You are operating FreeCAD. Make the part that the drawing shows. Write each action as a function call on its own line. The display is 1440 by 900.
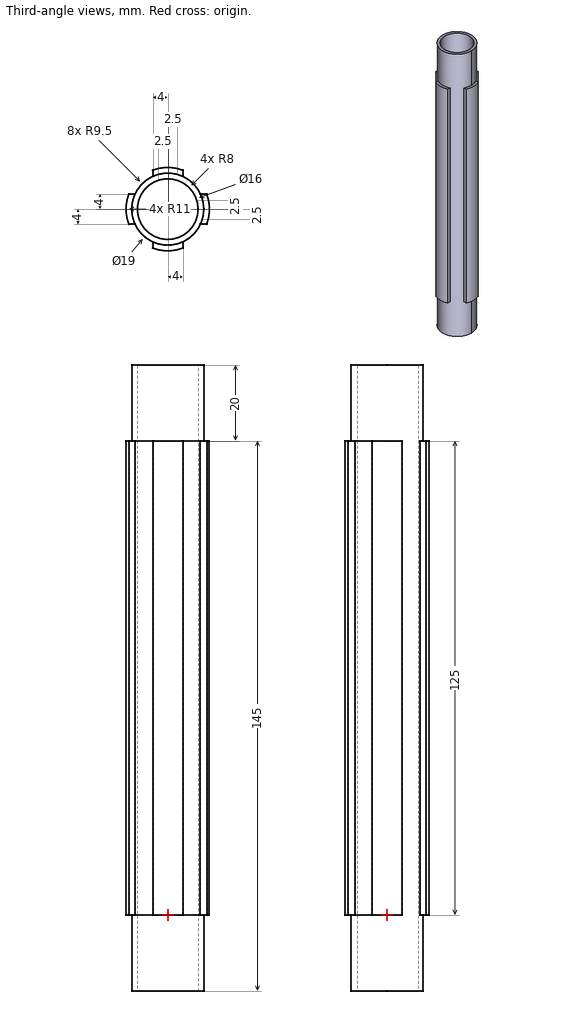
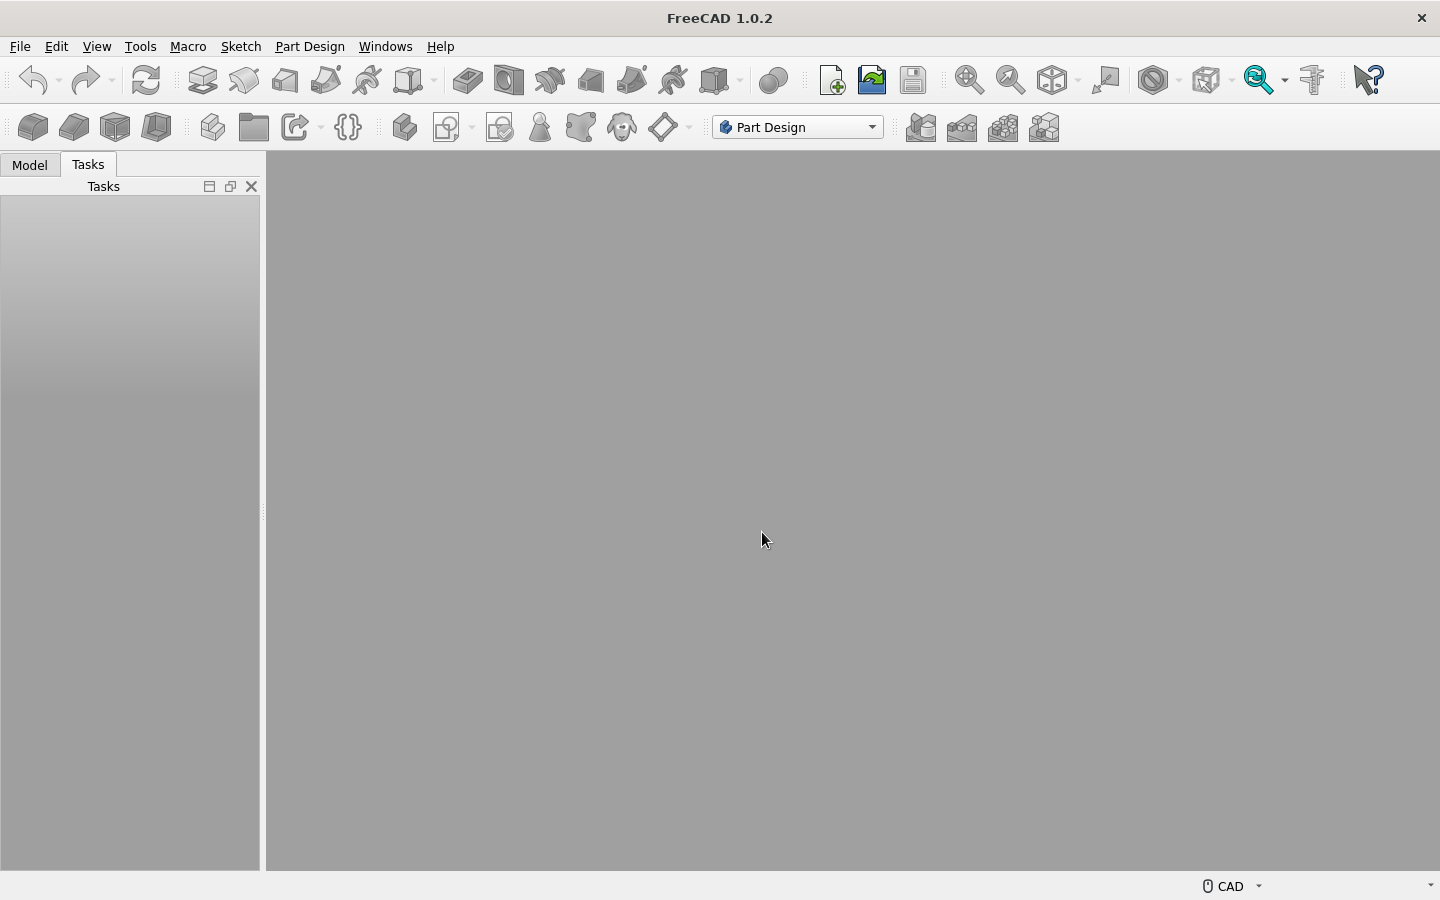
click(831, 80)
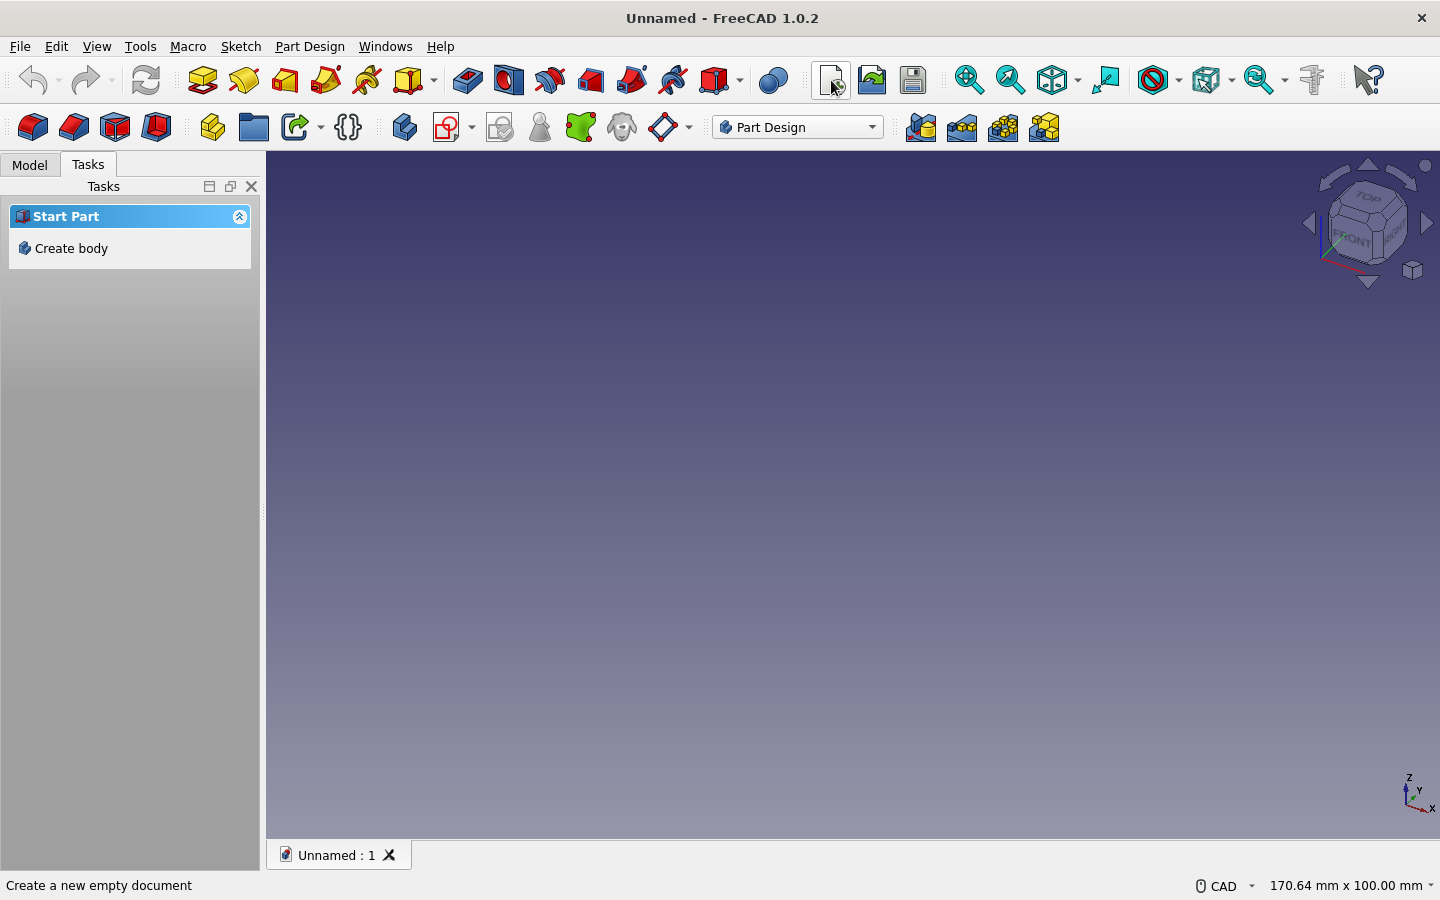
click(446, 128)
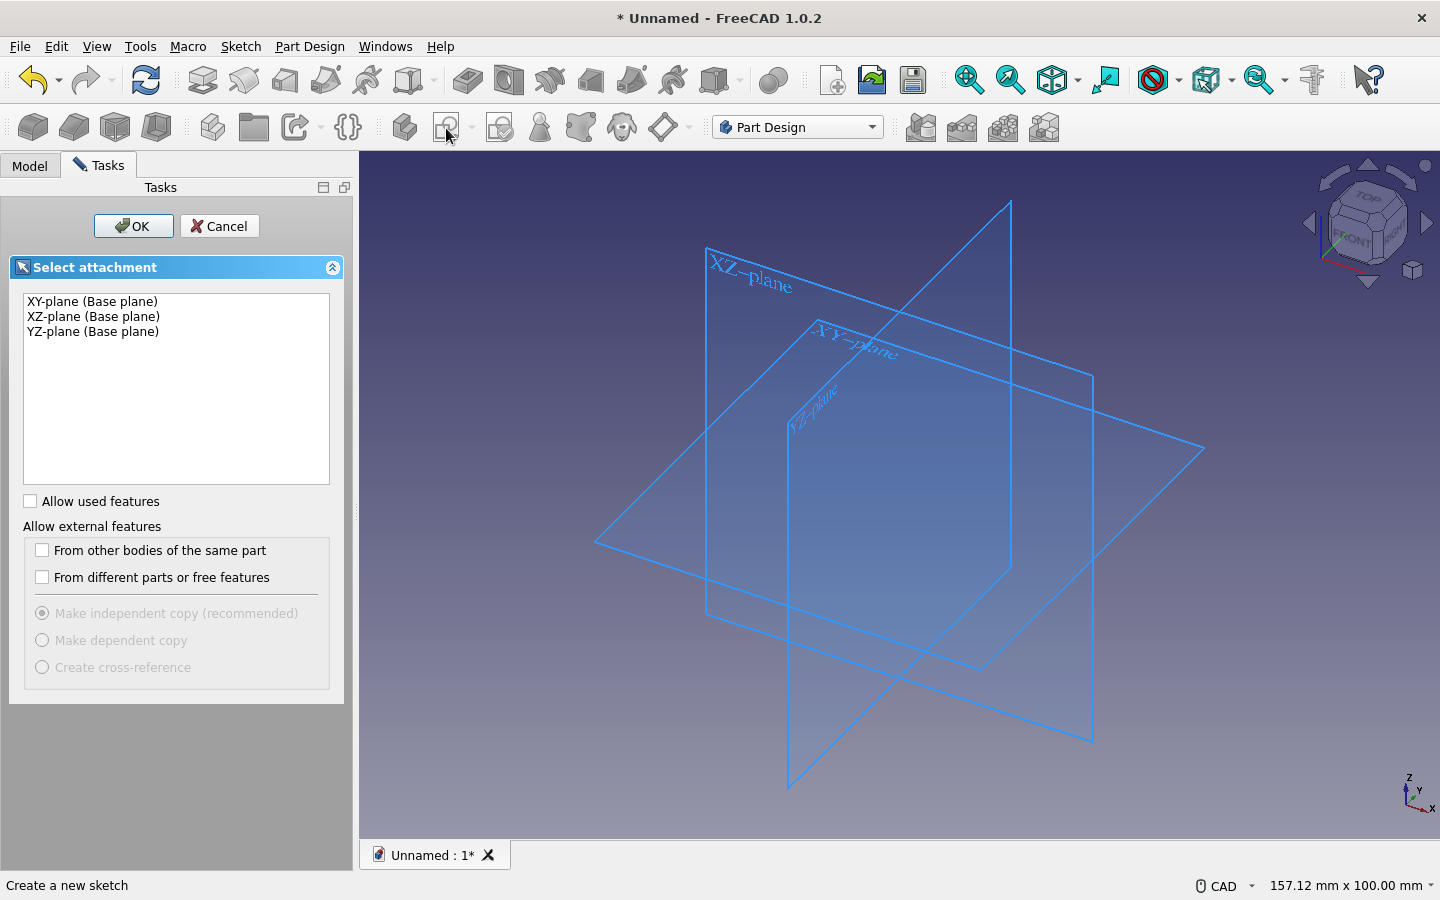
click(84, 302)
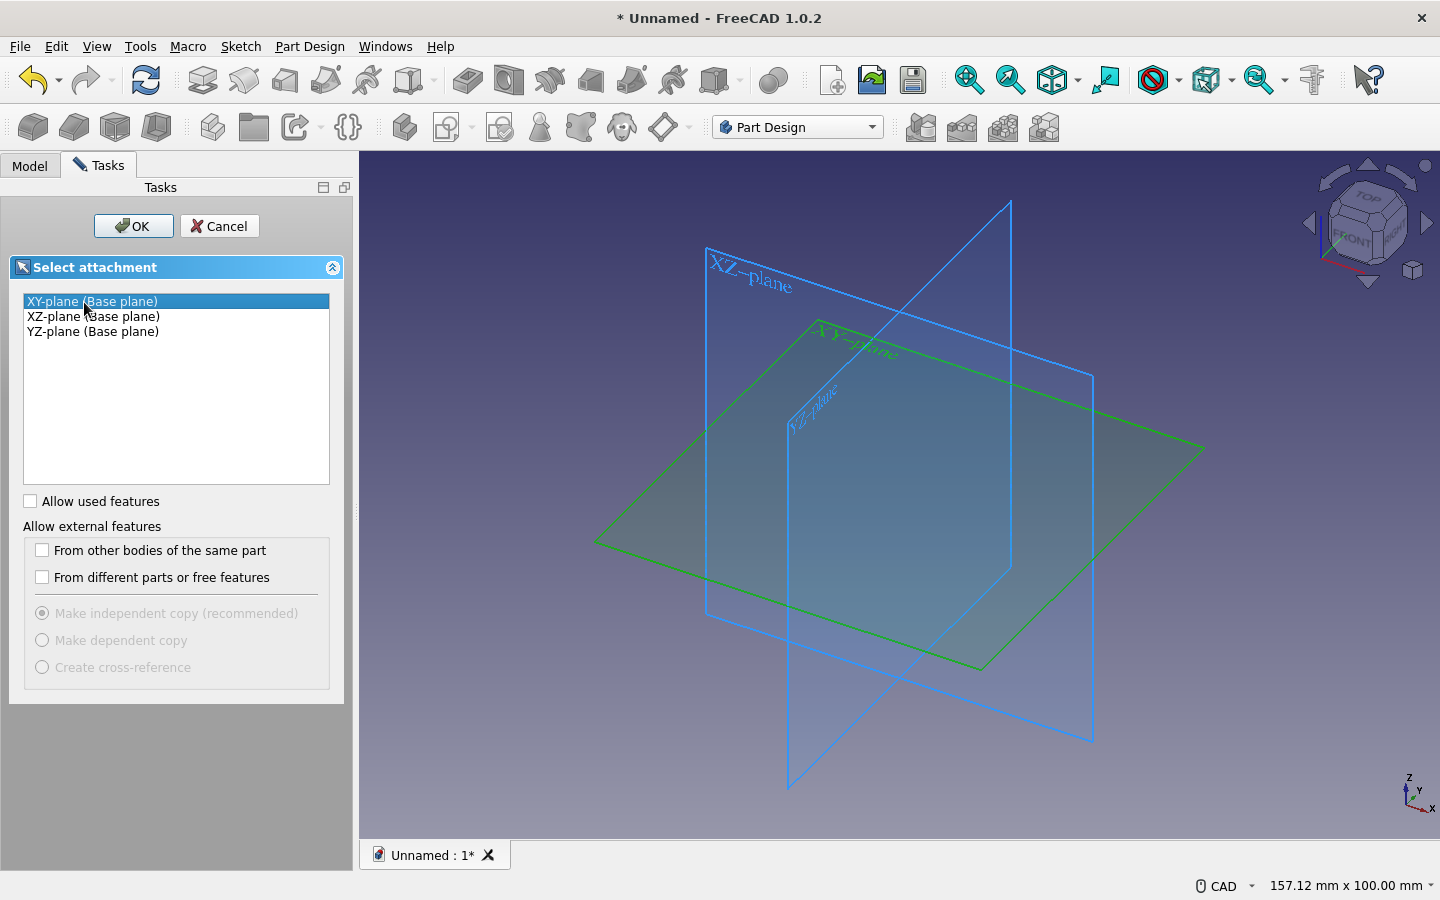
click(134, 226)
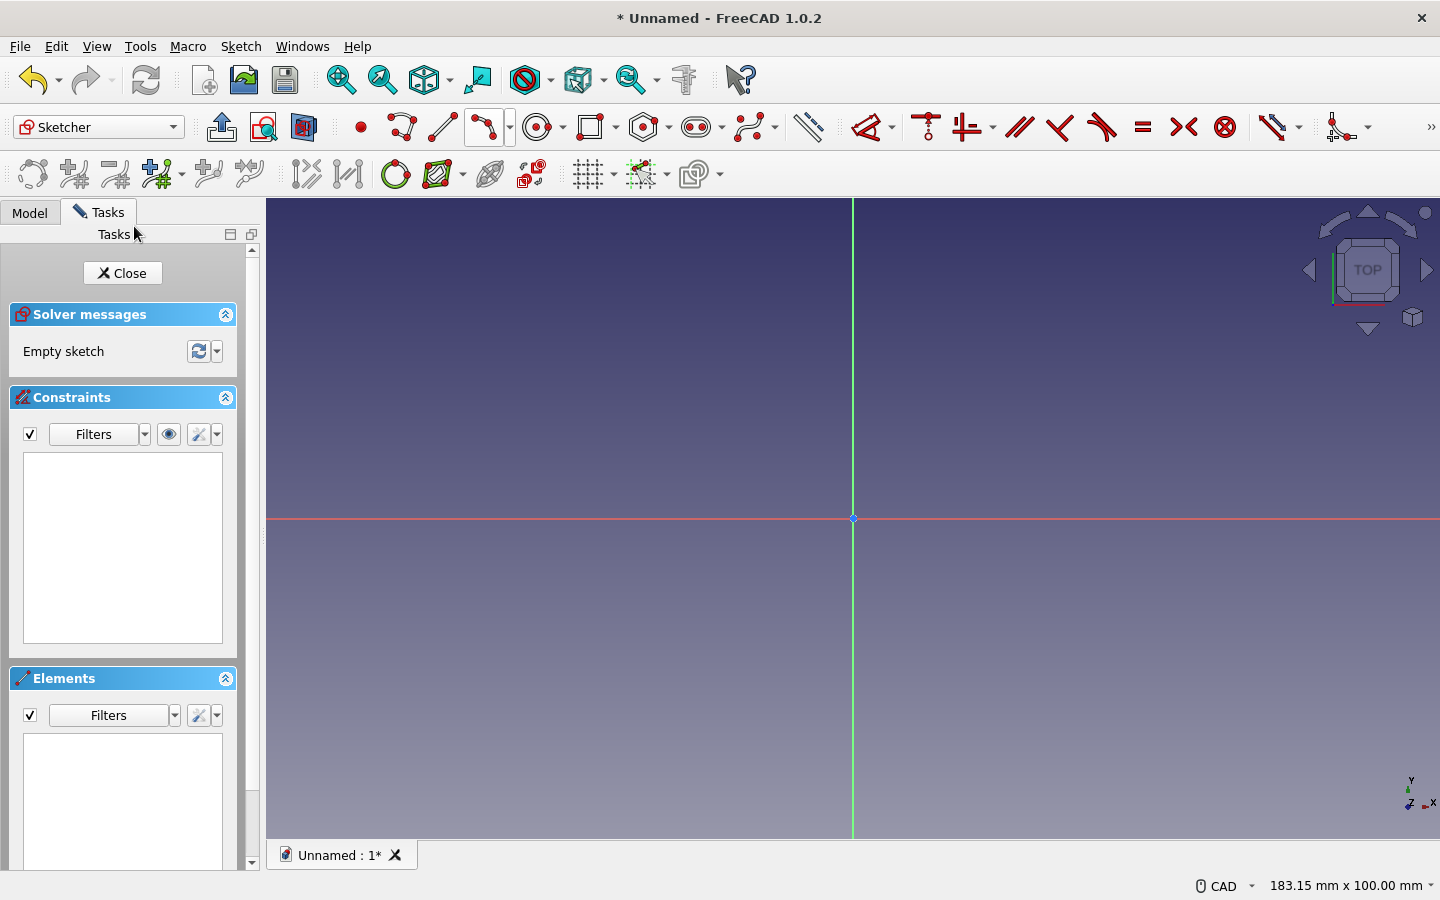
scroll(893, 518, up, 5)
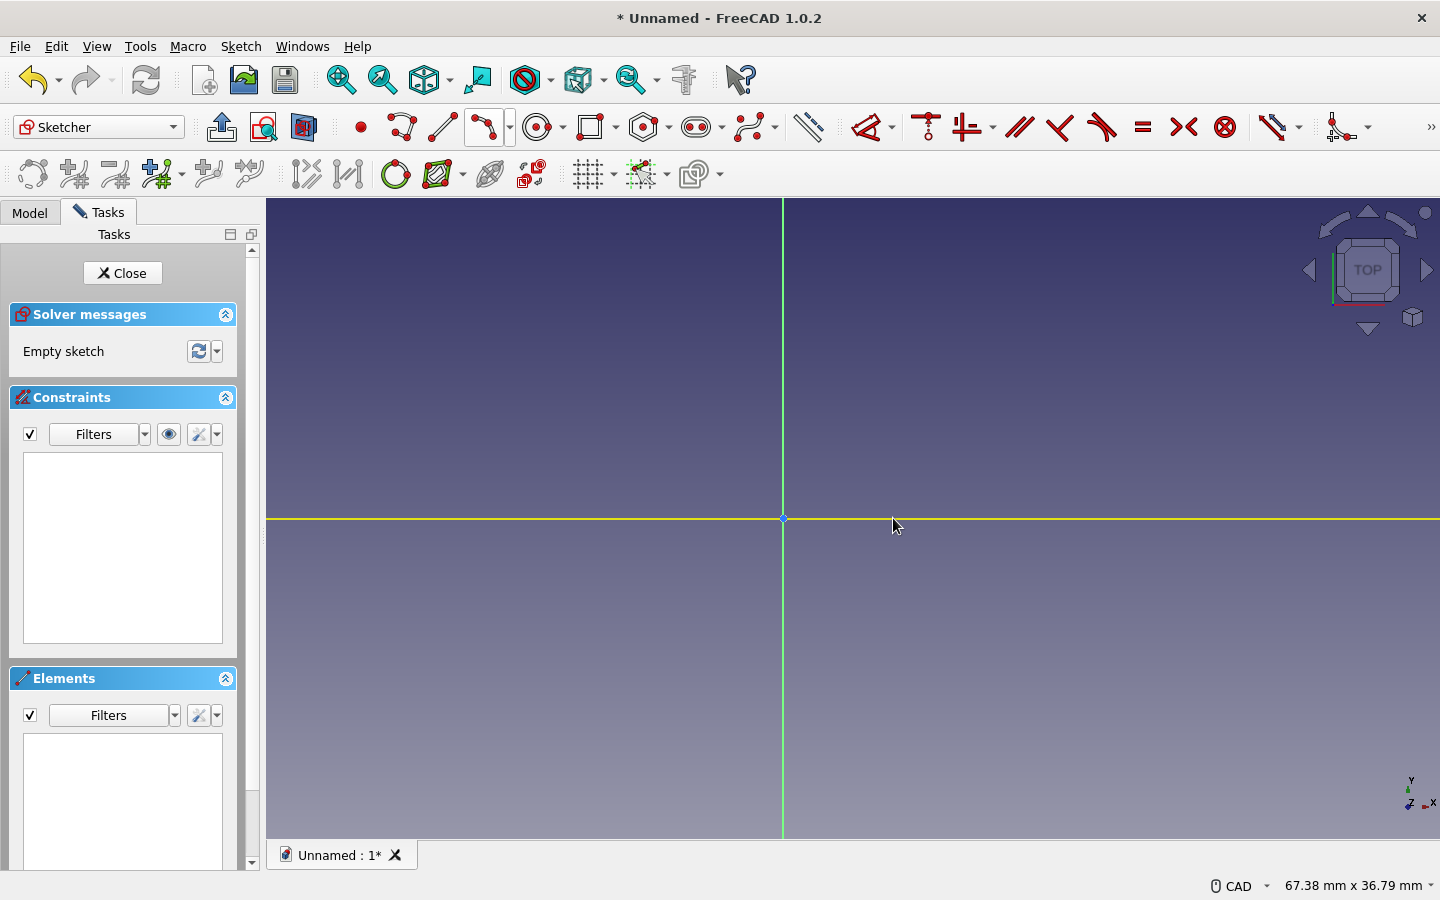
click(443, 128)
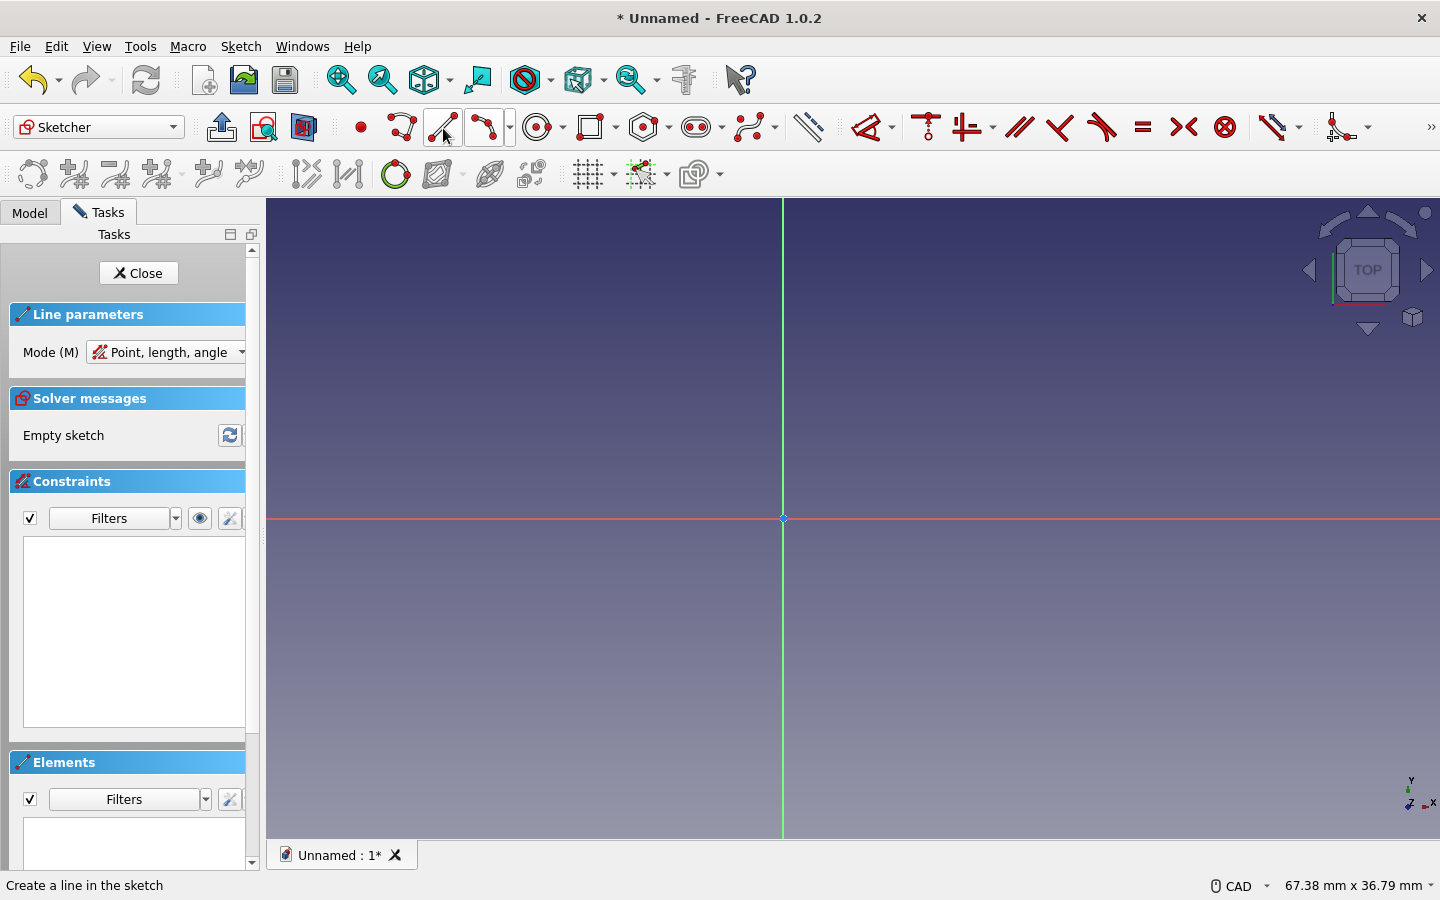
click(714, 340)
click(714, 368)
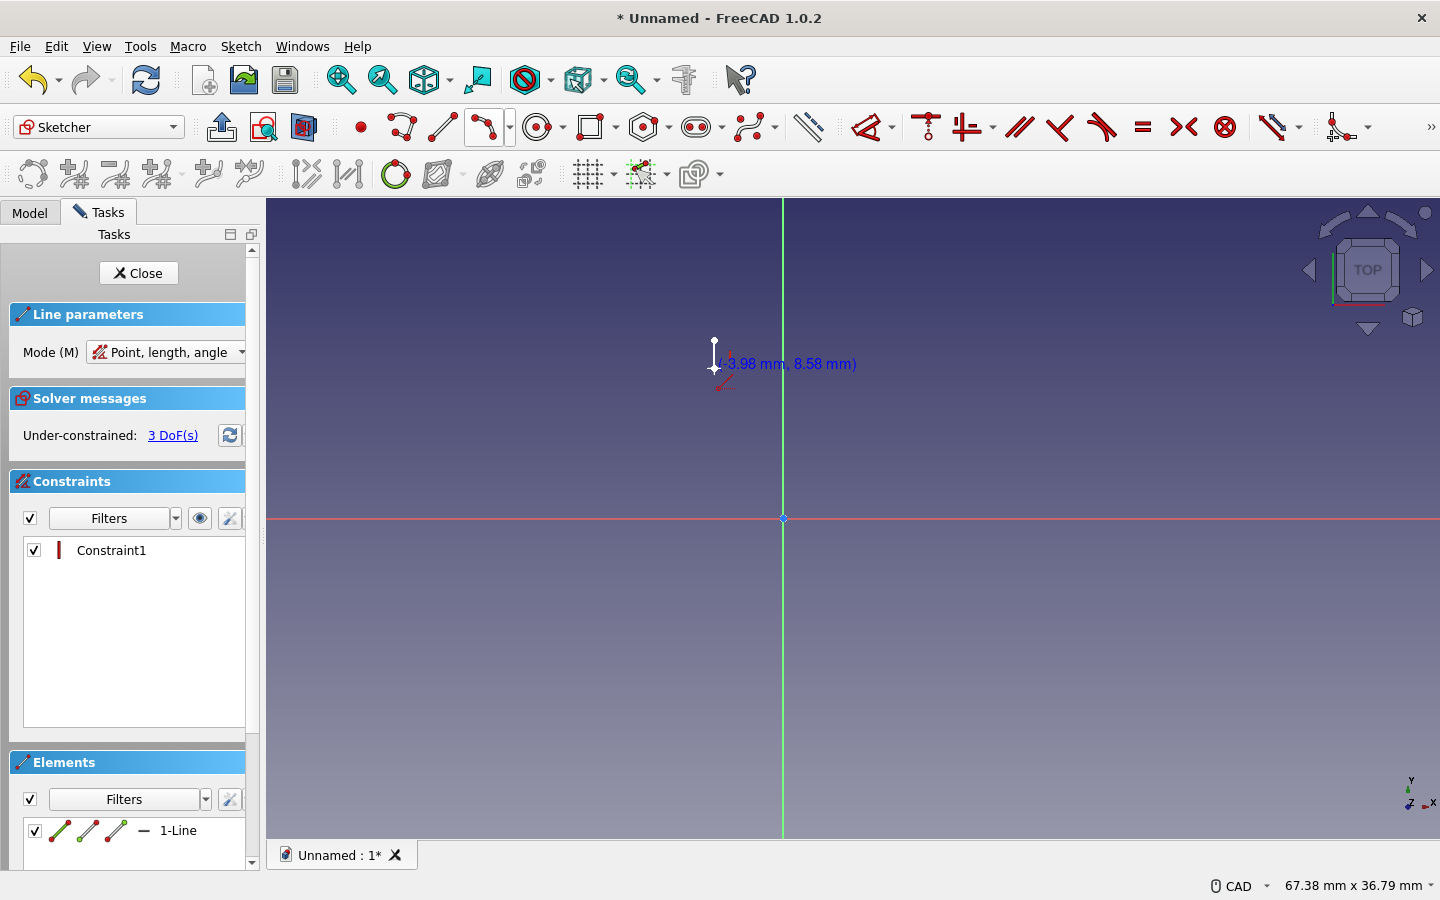
click(633, 449)
click(605, 449)